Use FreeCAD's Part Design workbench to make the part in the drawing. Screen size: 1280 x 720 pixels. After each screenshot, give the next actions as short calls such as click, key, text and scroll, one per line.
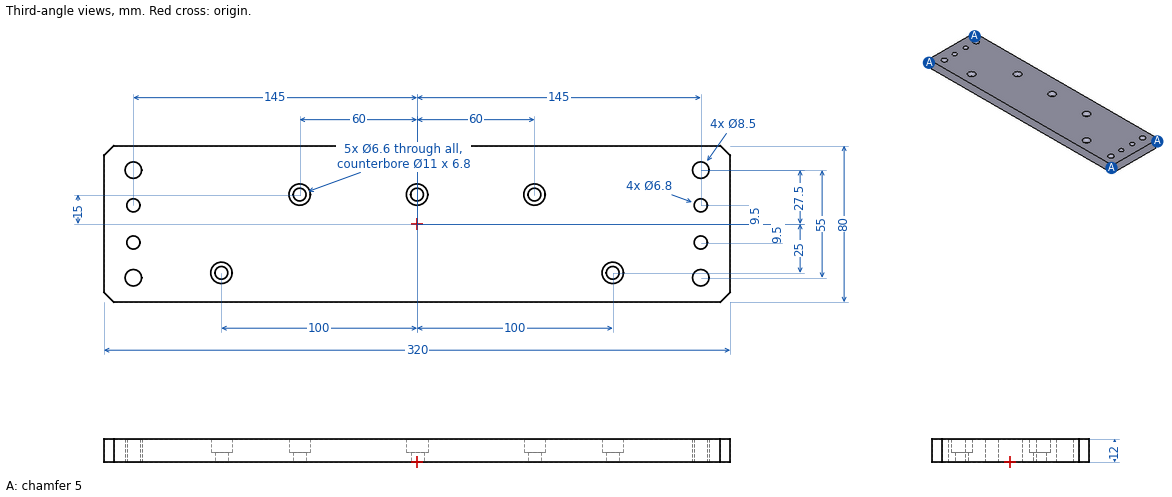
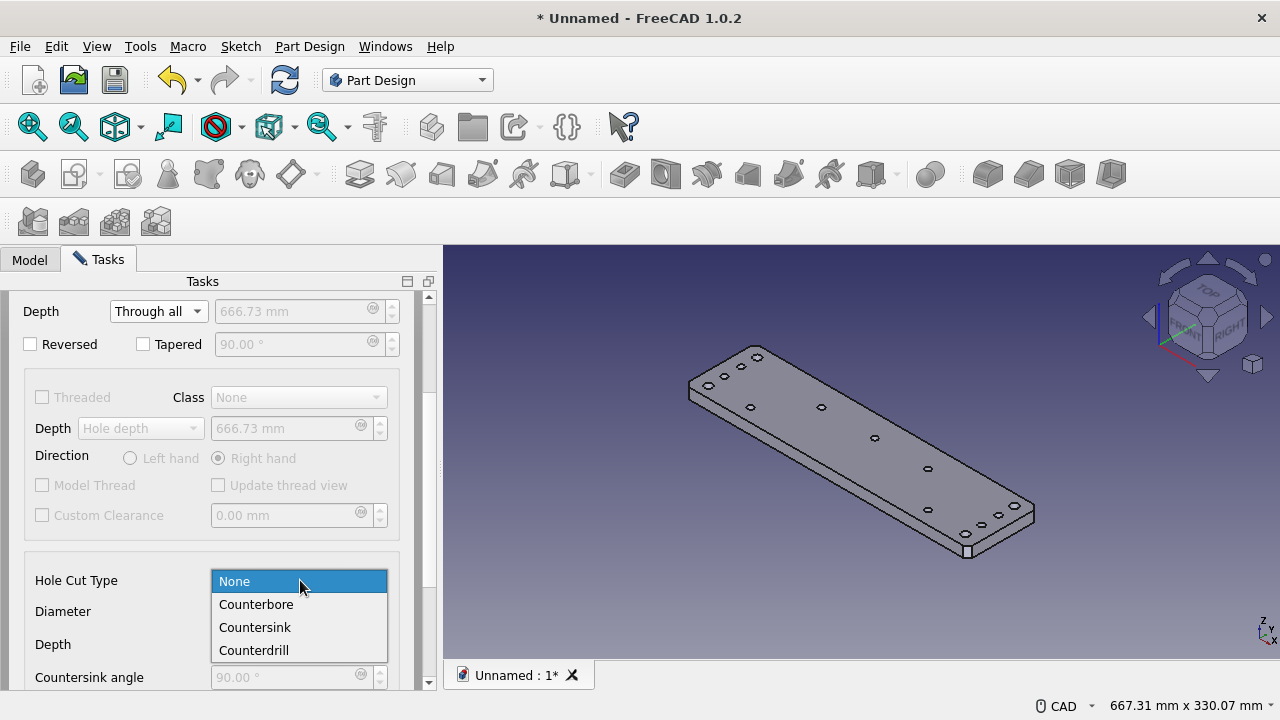
click(298, 604)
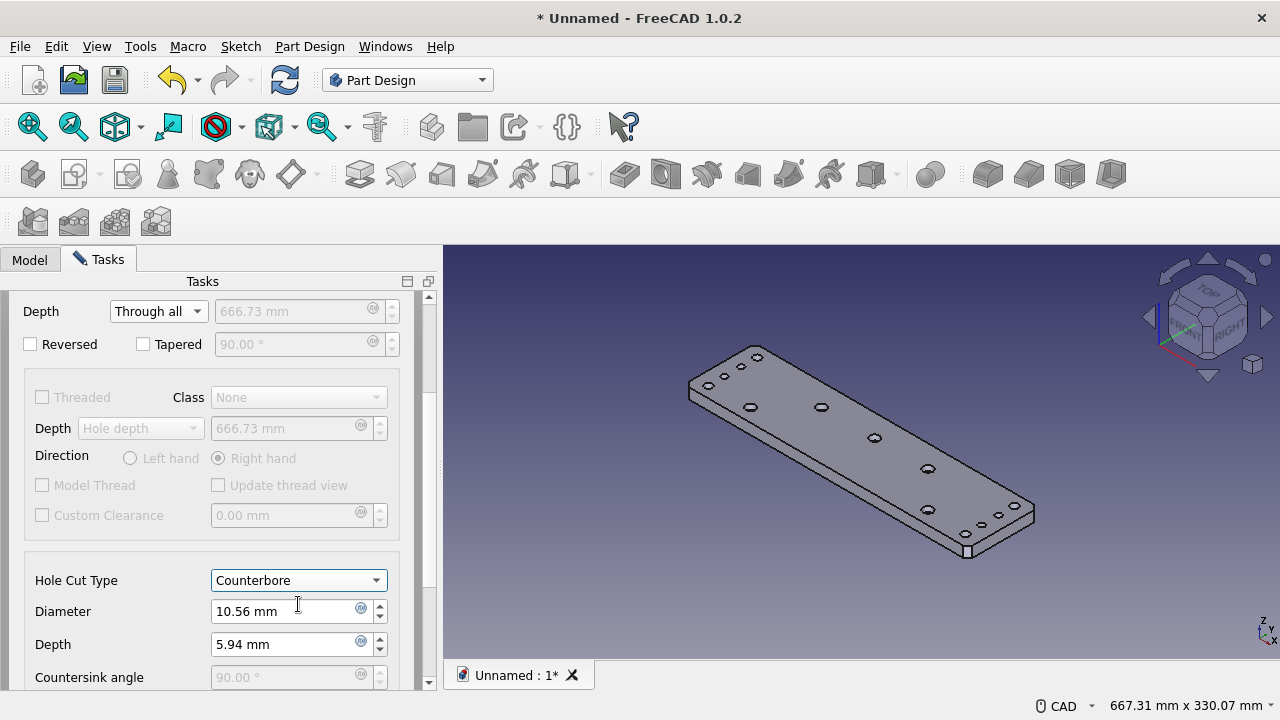
triple_click(292, 612)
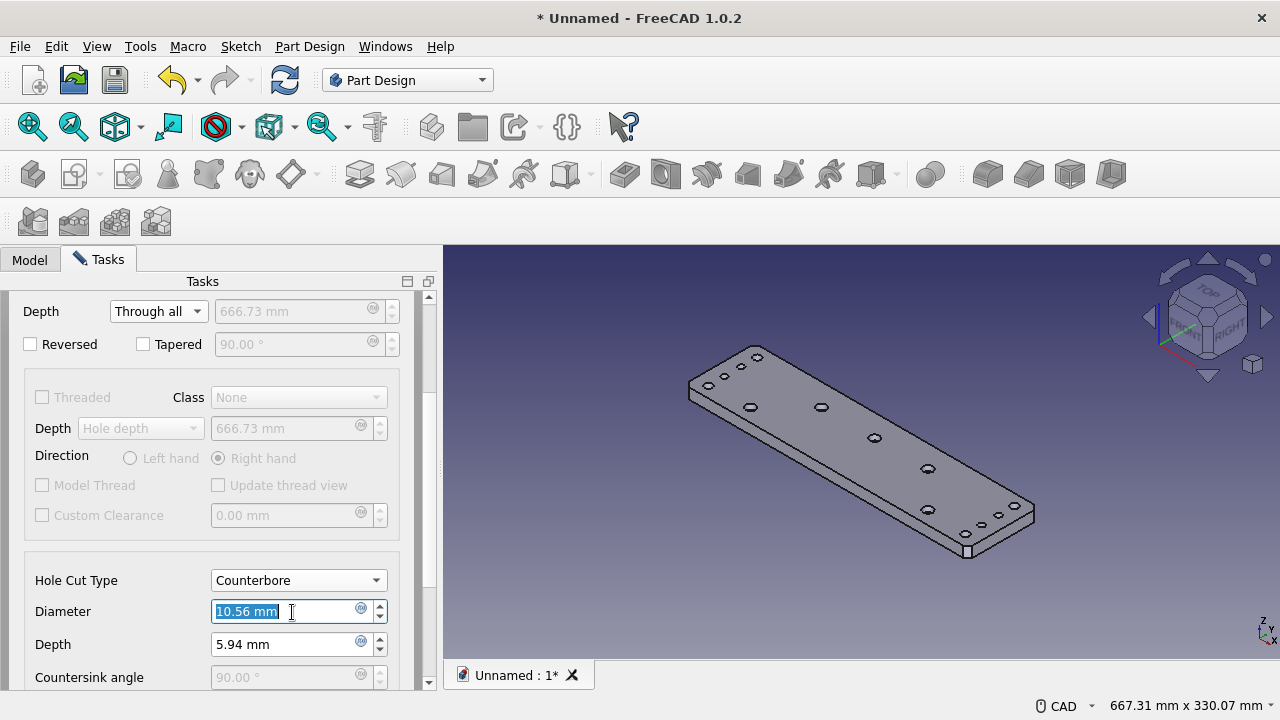
text(11)
key(Tab)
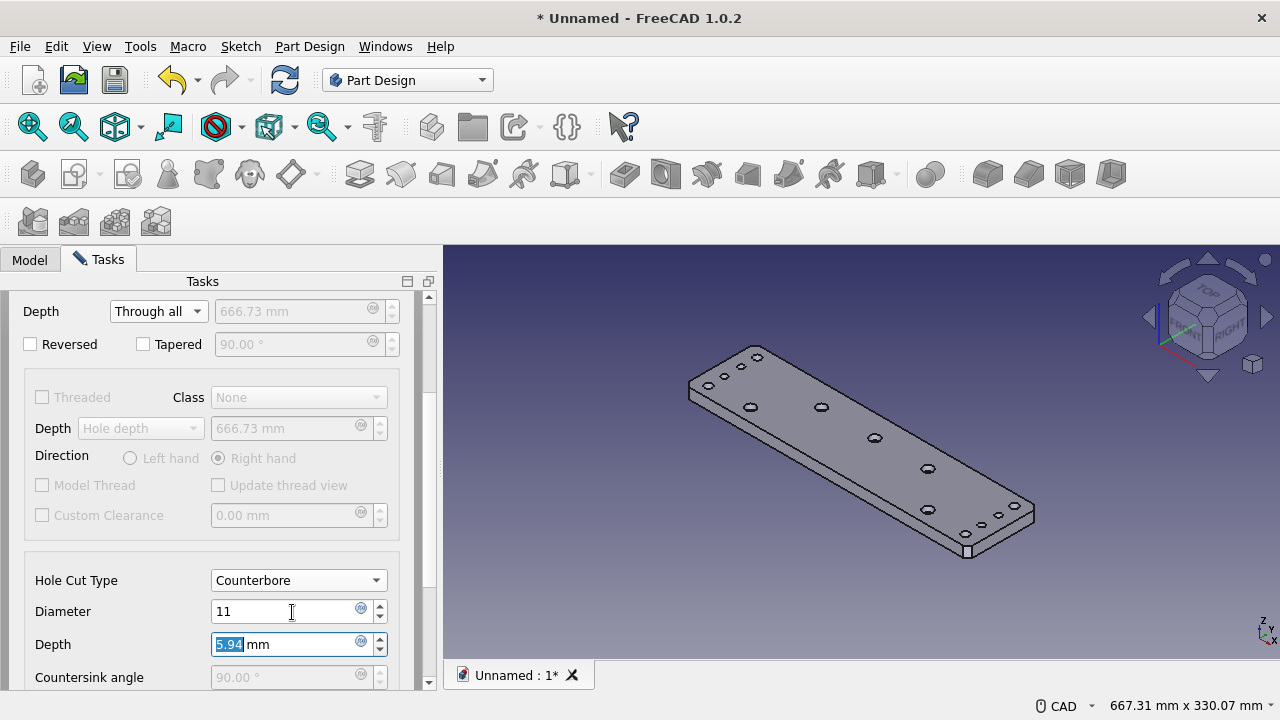
text(6.8)
key(Tab)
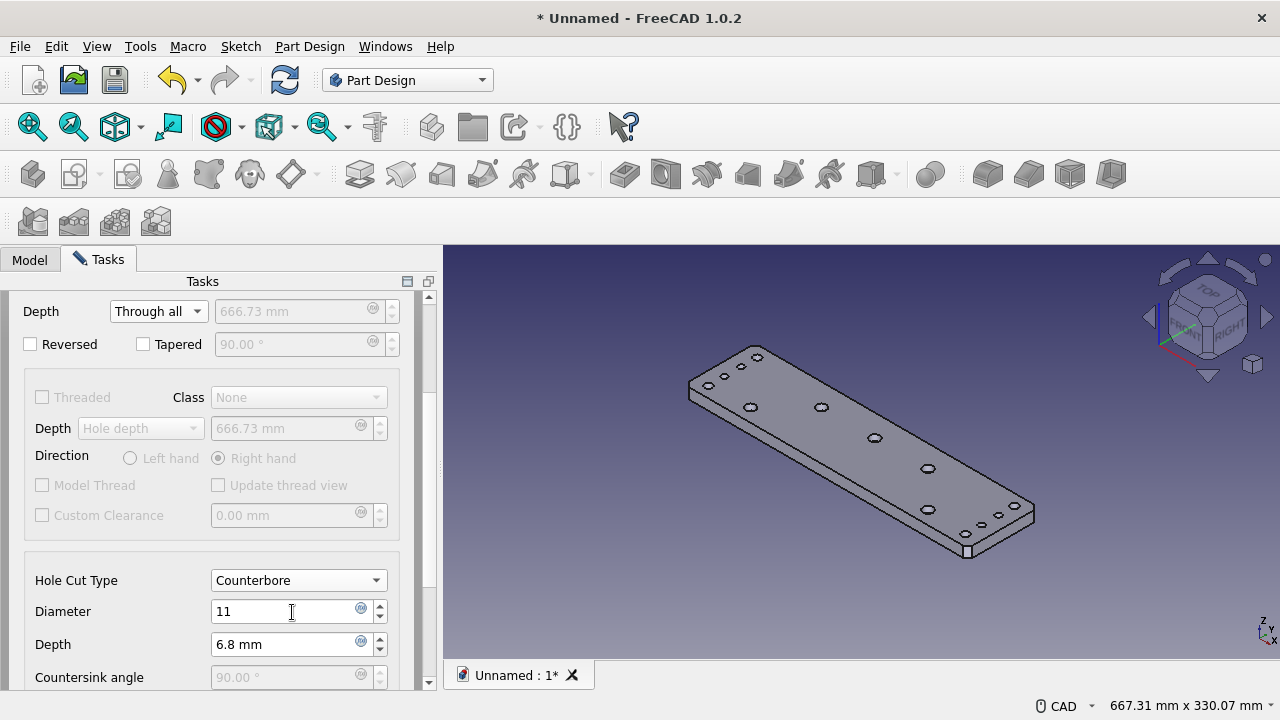
scroll(429, 490, up, 4)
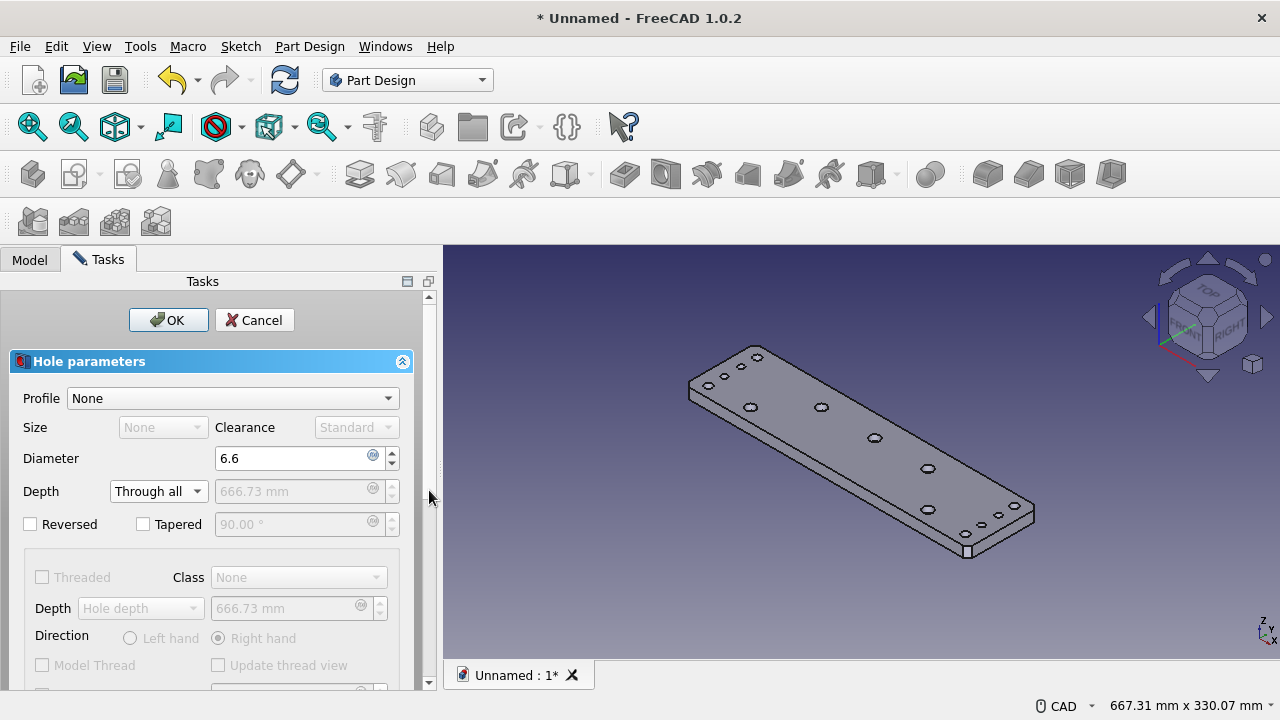
click(169, 320)